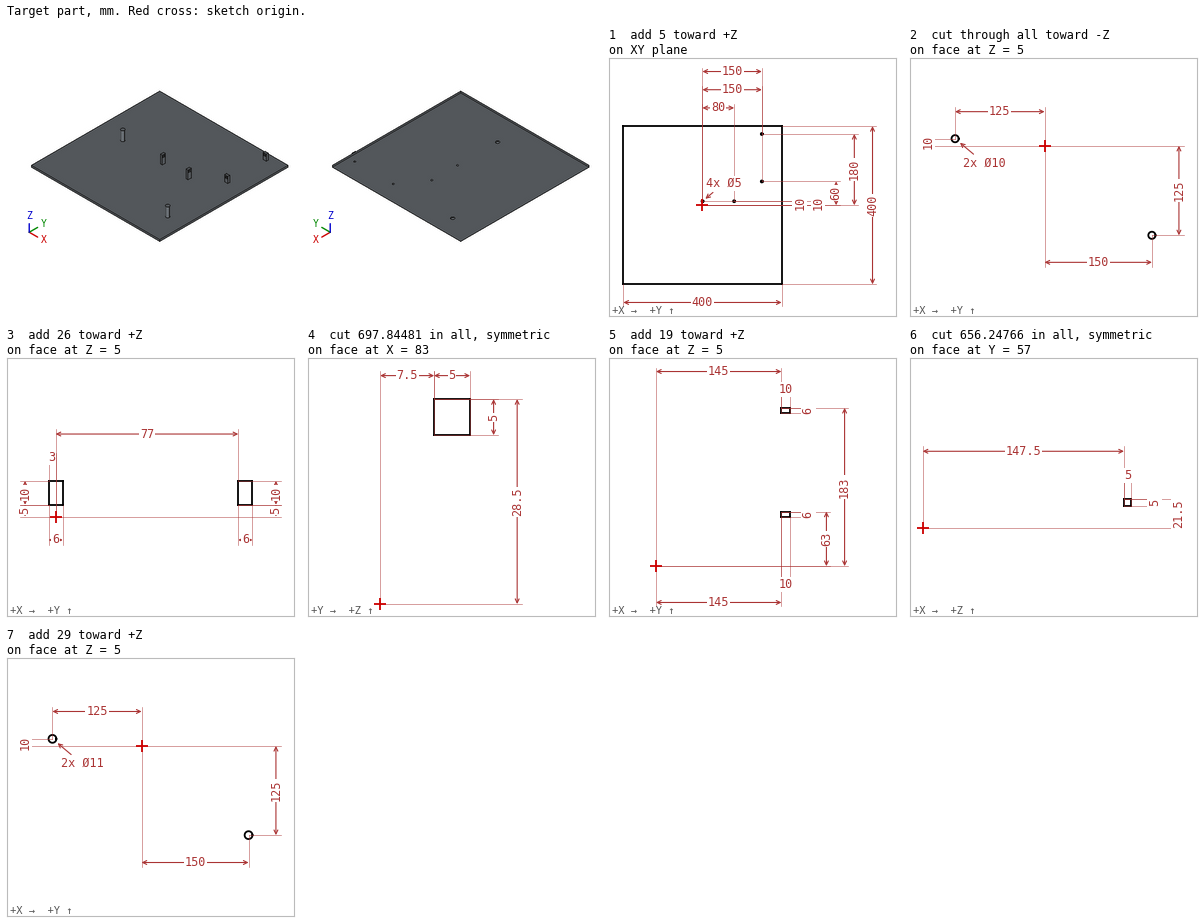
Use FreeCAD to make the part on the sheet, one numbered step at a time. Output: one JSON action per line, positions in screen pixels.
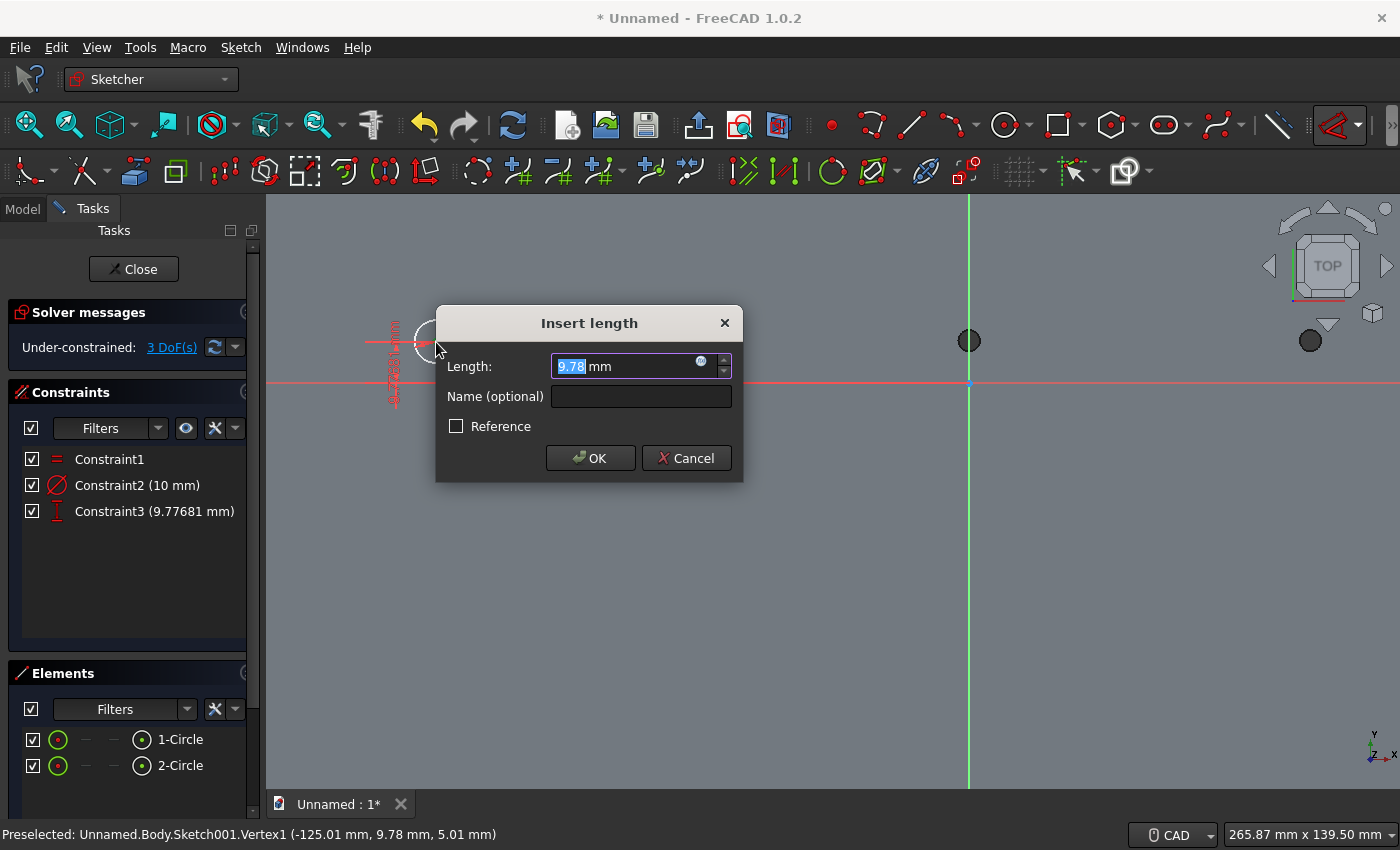
{"action": "type", "text": "10"}
{"action": "key", "text": "Return"}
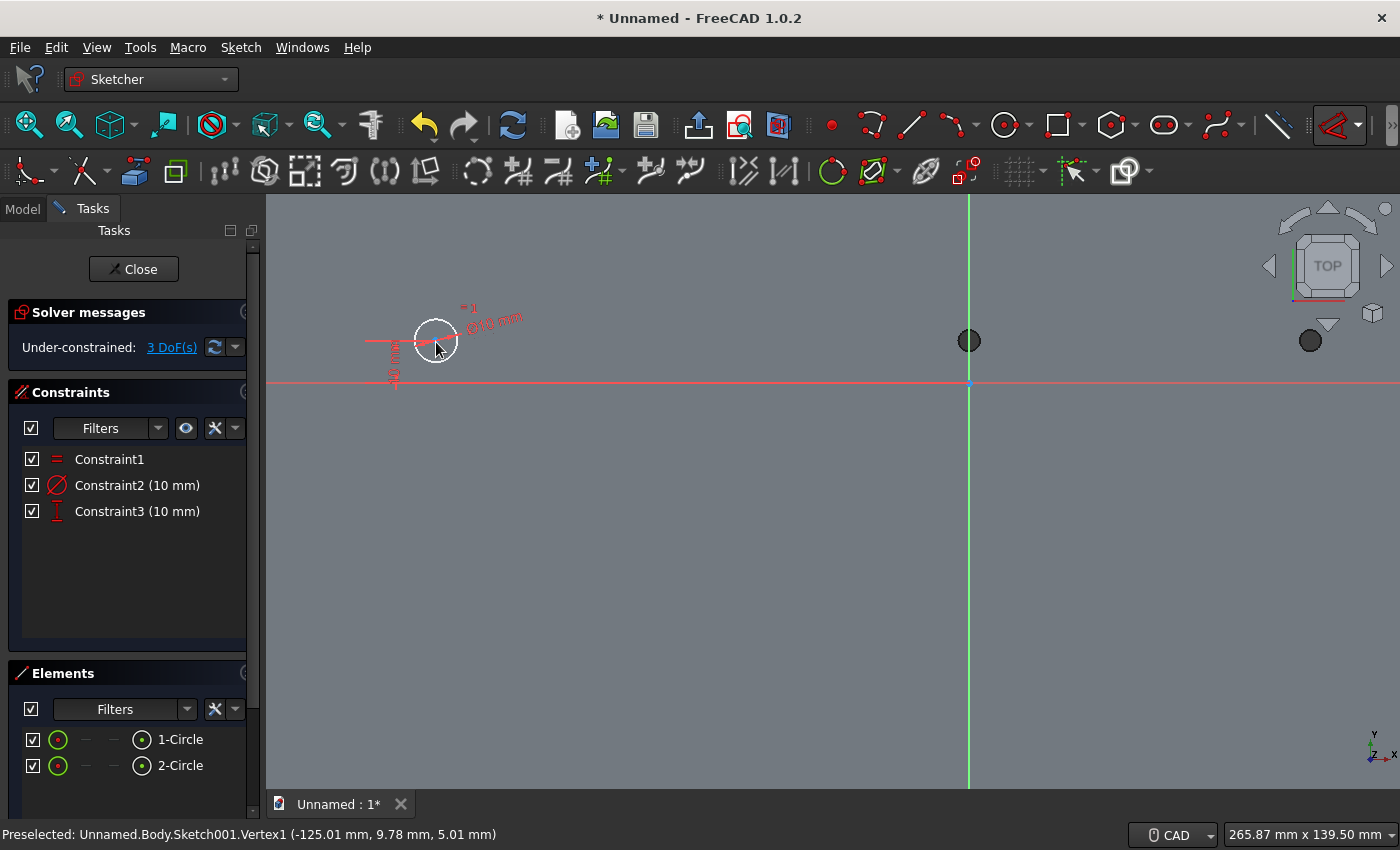
{"action": "left_click", "coordinate": [436, 341]}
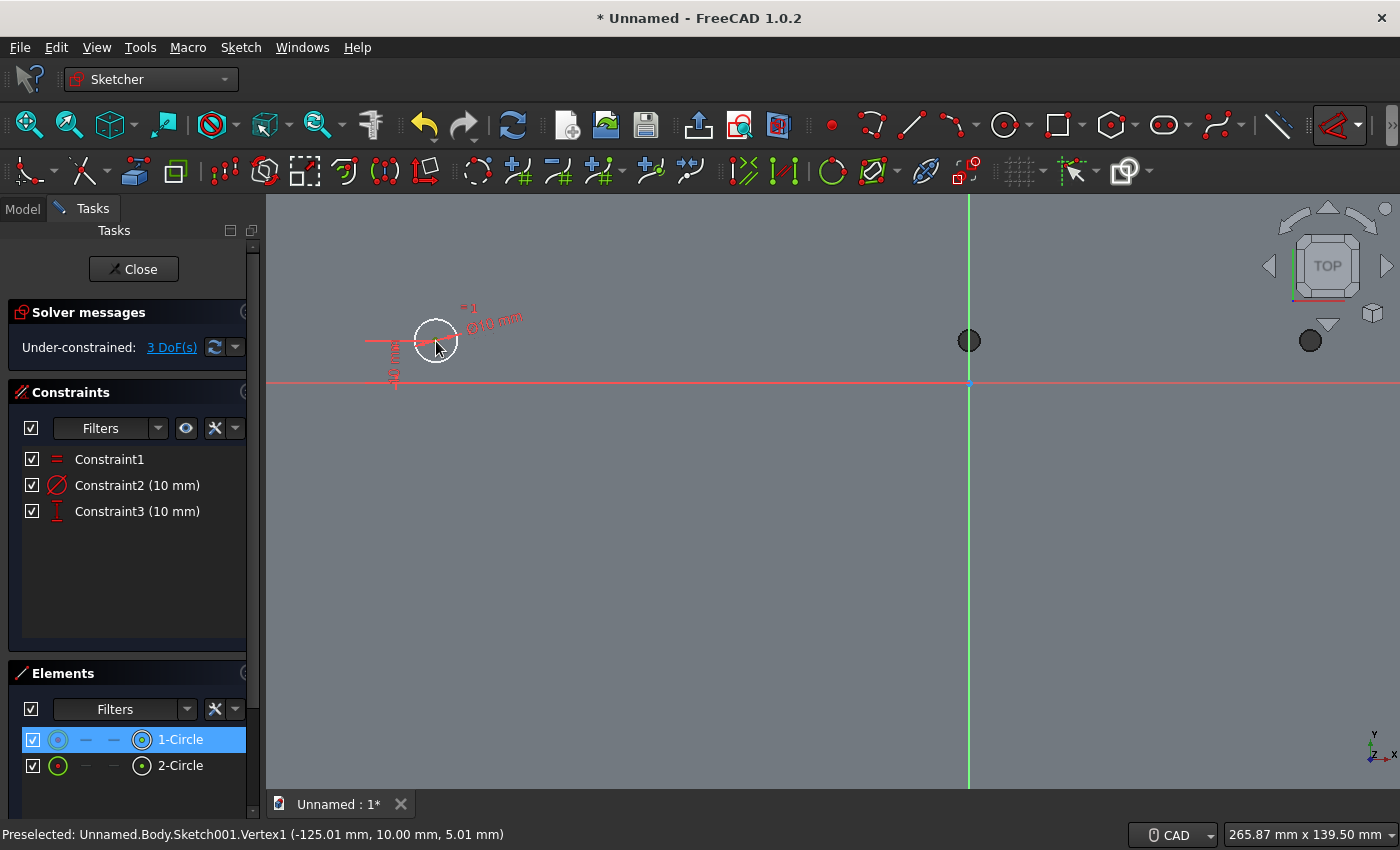
{"action": "key", "text": "l"}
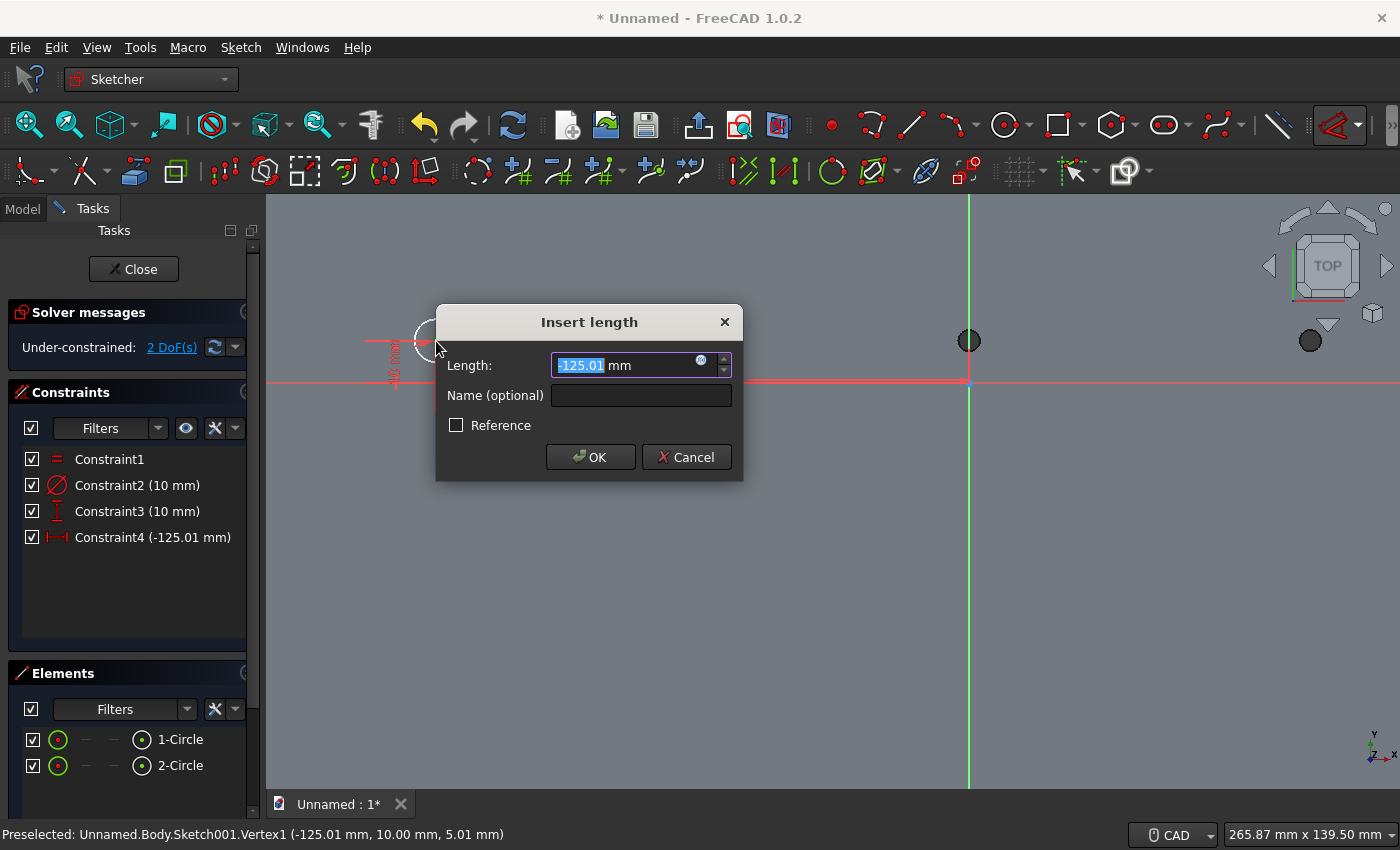
{"action": "type", "text": "-125"}
{"action": "key", "text": "Return"}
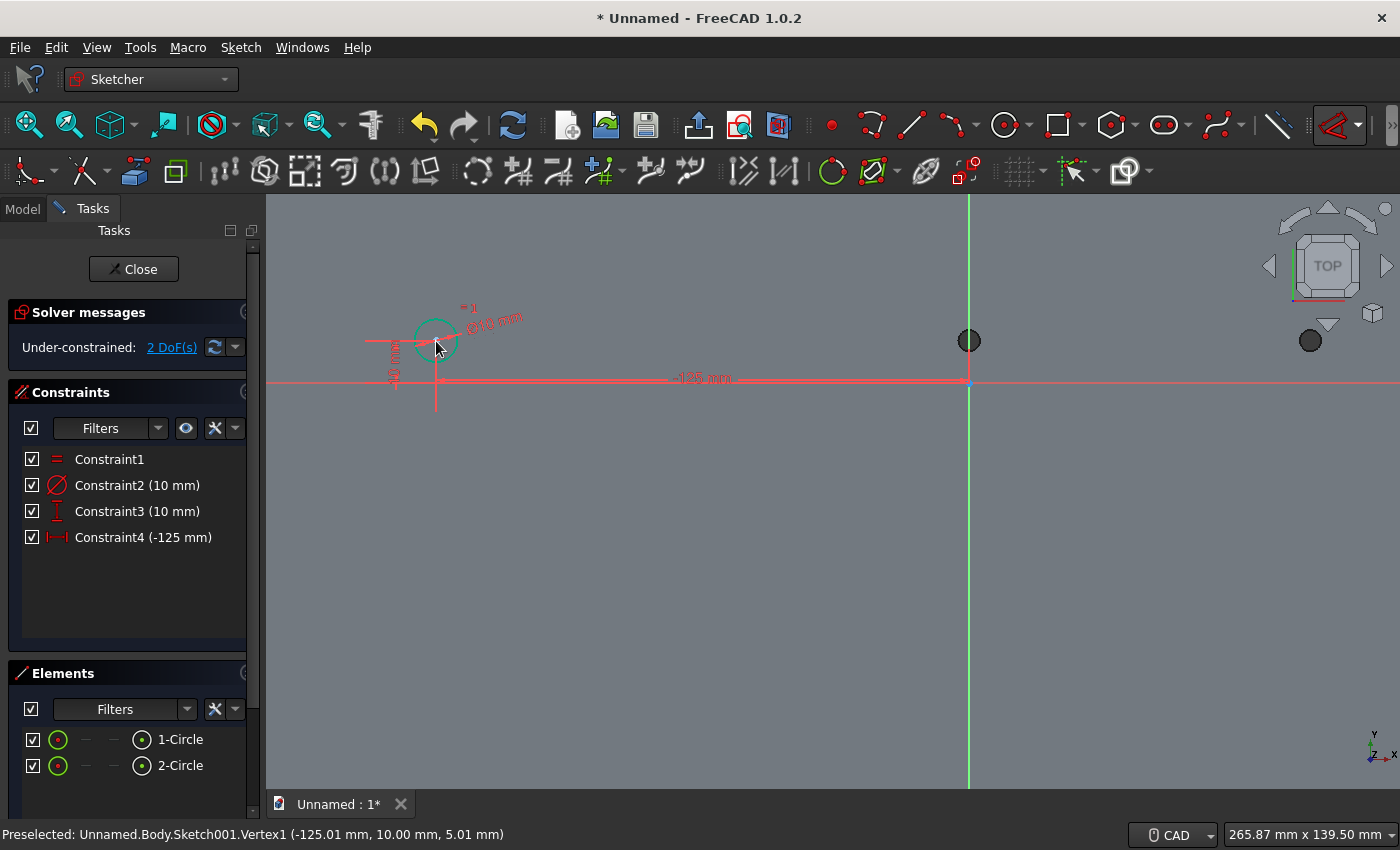
{"action": "scroll", "coordinate": [451, 325], "scroll_direction": "down", "scroll_amount": 3}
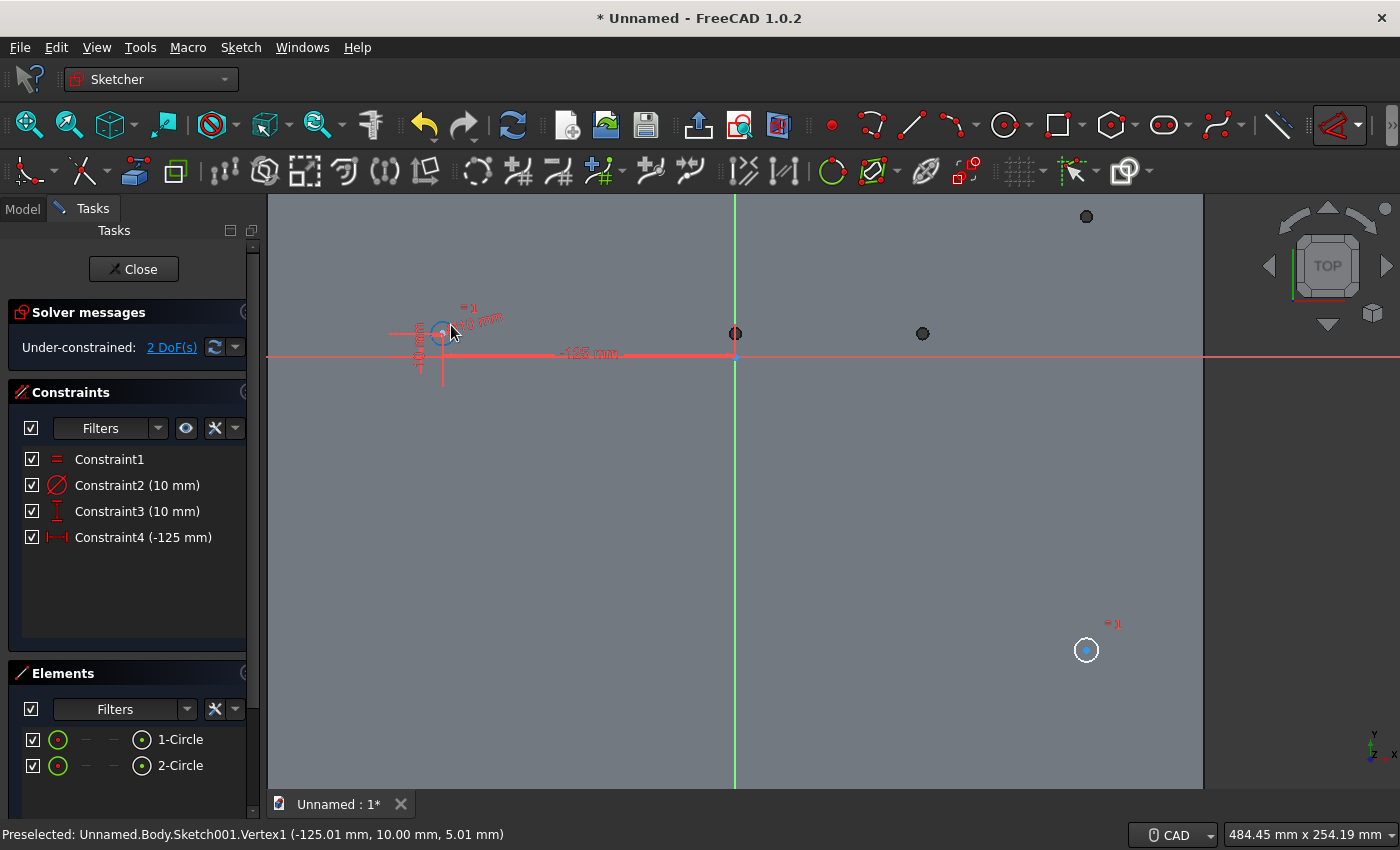
{"action": "left_click", "coordinate": [1086, 650]}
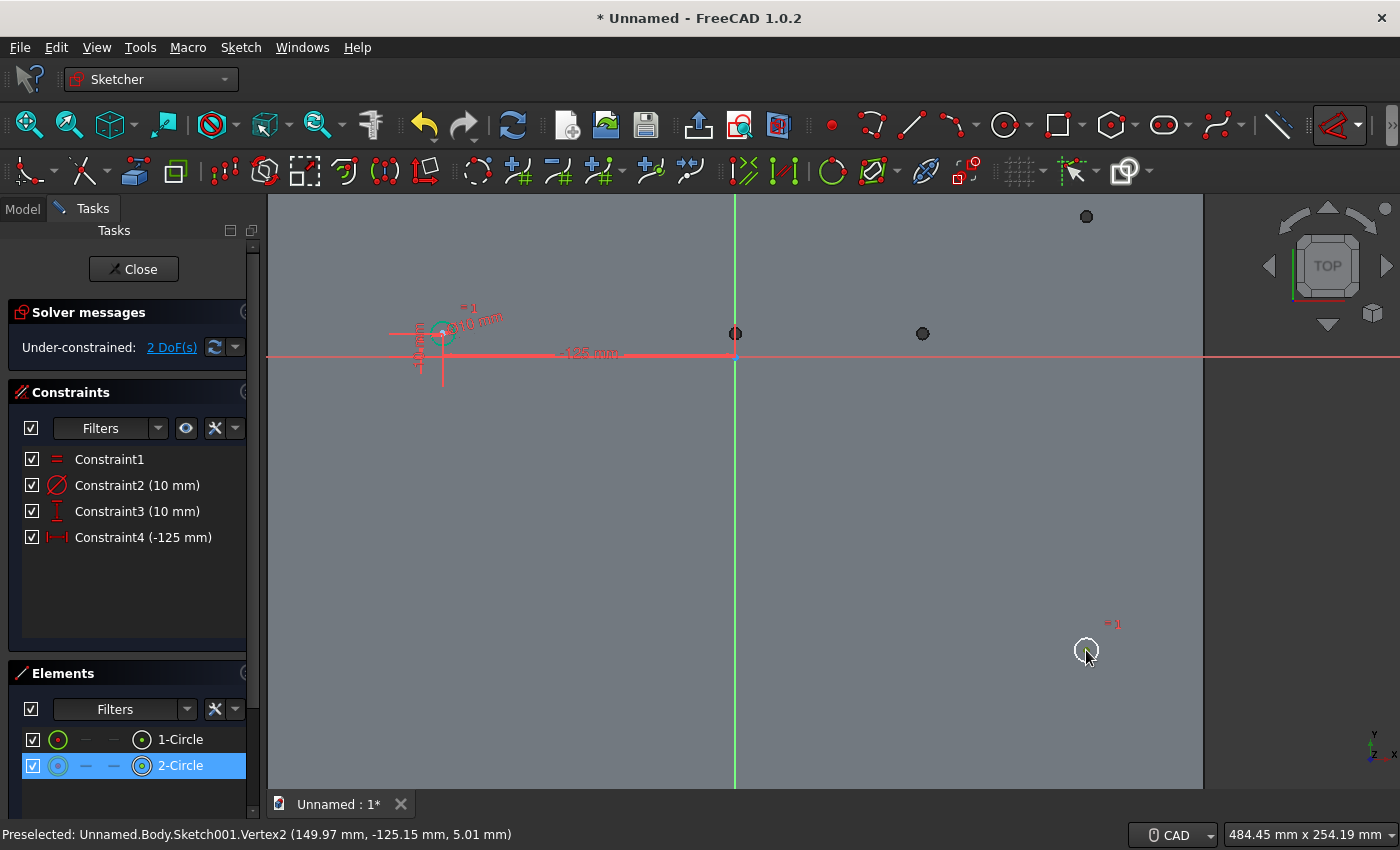
{"action": "key", "text": "l"}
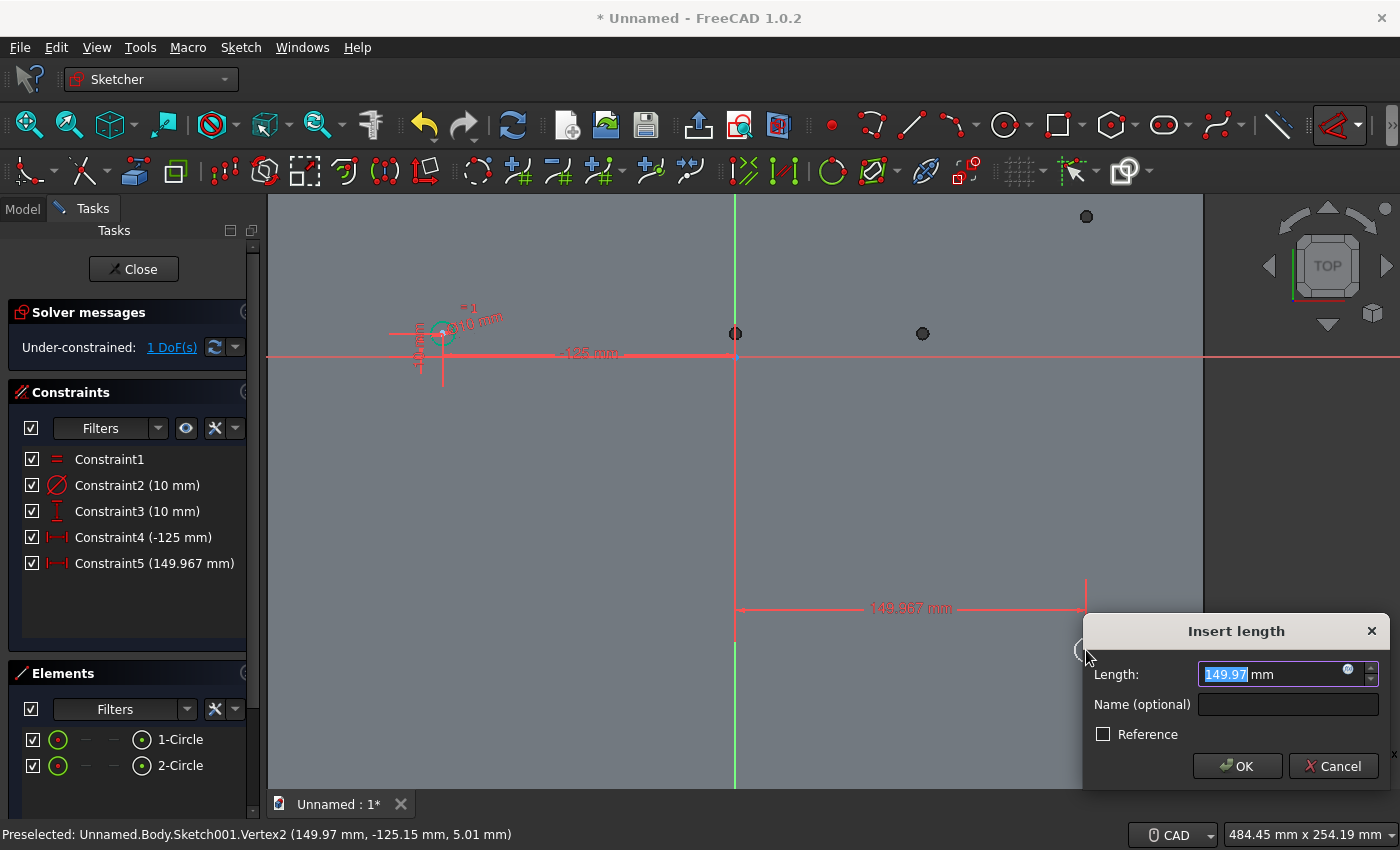
{"action": "type", "text": "150"}
{"action": "key", "text": "Return"}